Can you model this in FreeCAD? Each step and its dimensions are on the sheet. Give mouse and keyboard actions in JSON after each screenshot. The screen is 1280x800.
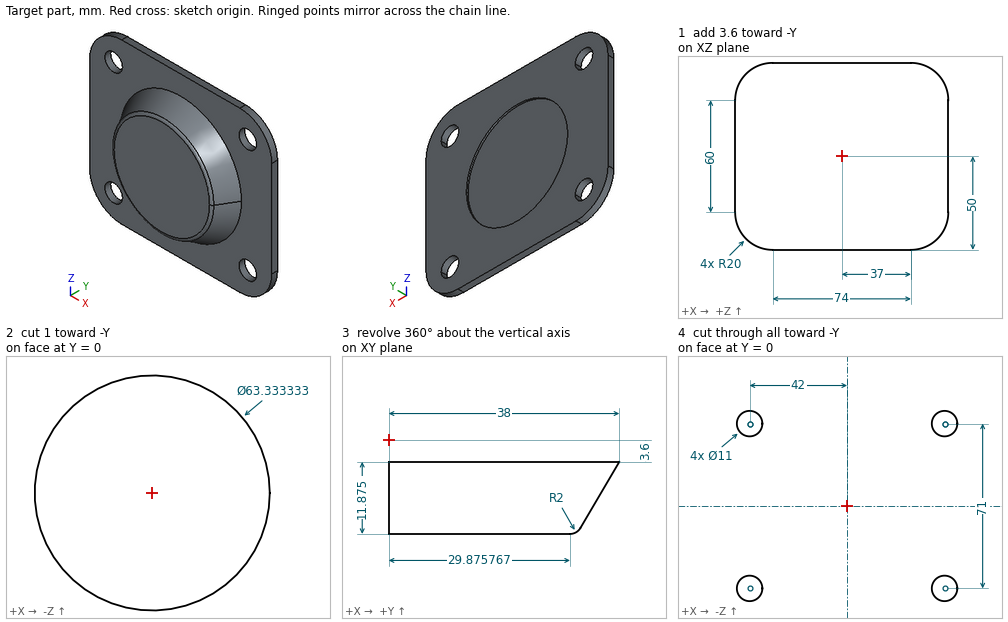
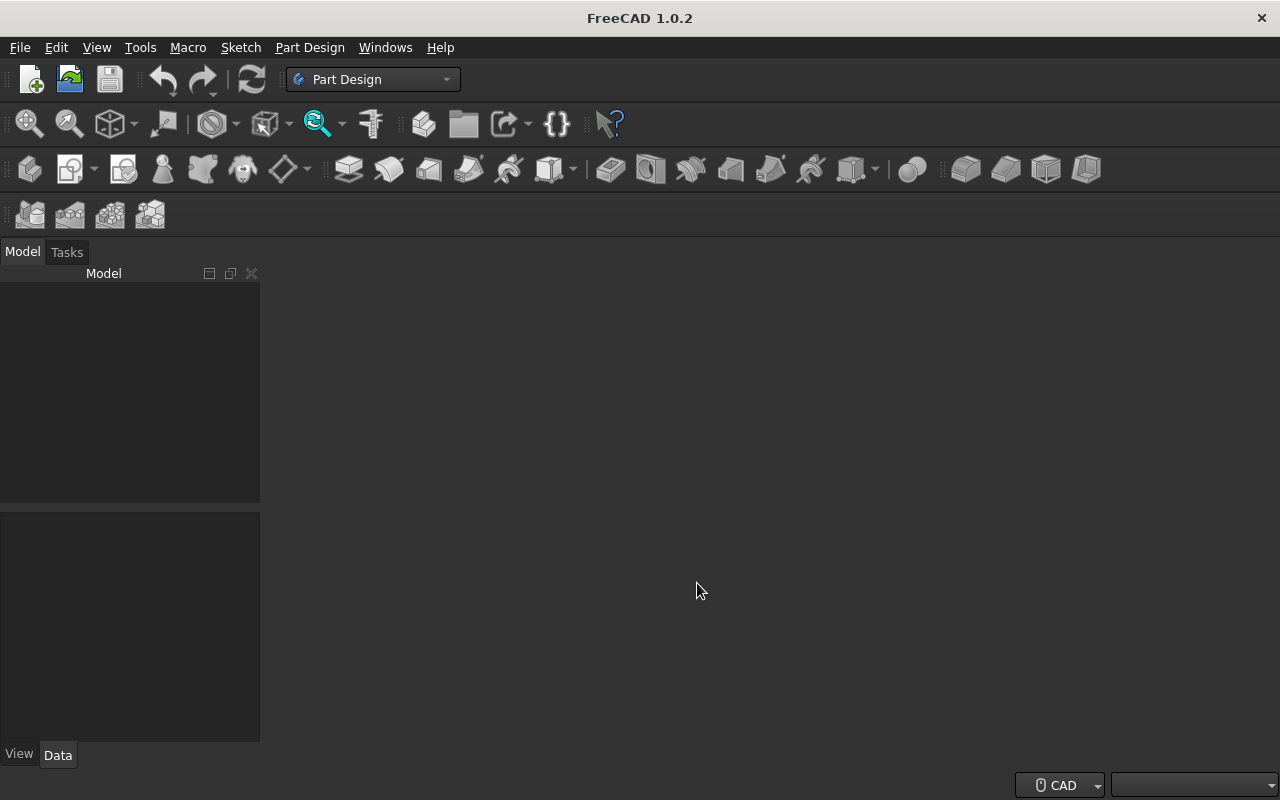
{"action": "left_click", "coordinate": [30, 80]}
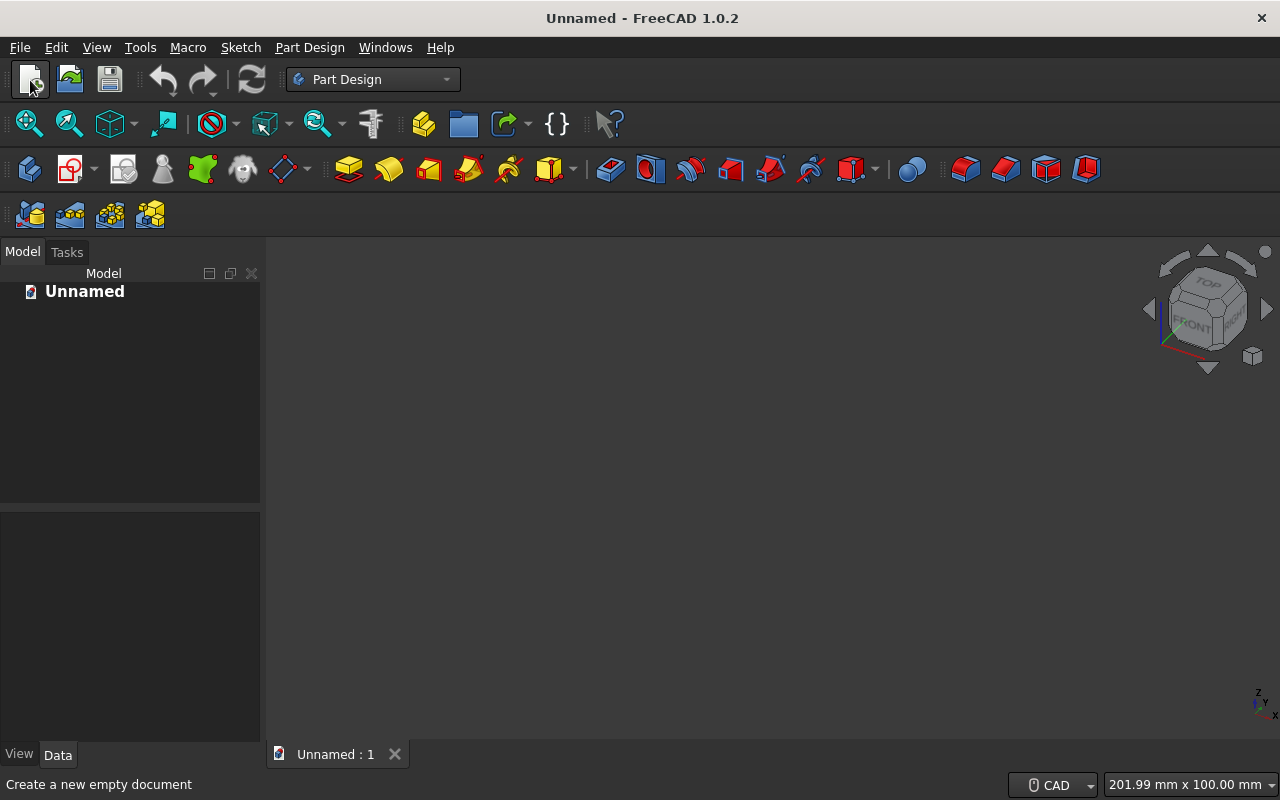
{"action": "left_click", "coordinate": [70, 170]}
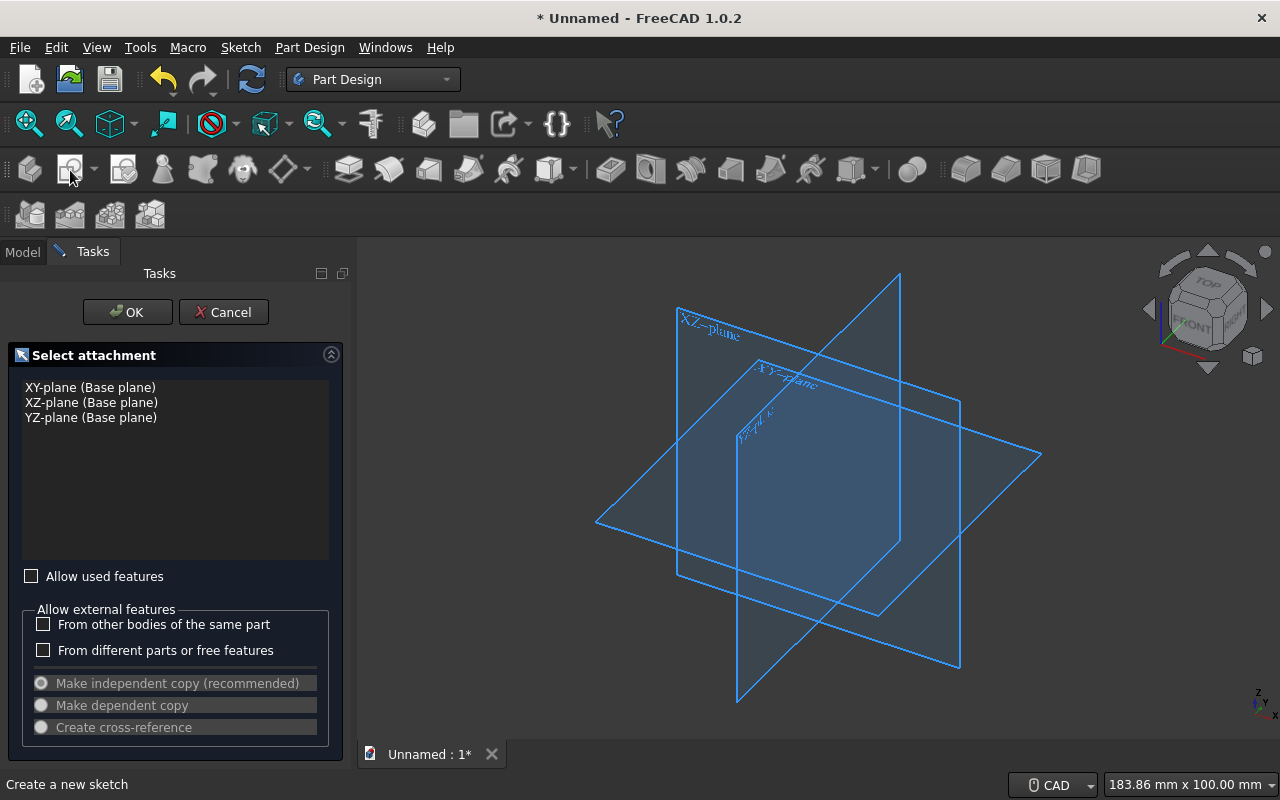
{"action": "left_click", "coordinate": [82, 402]}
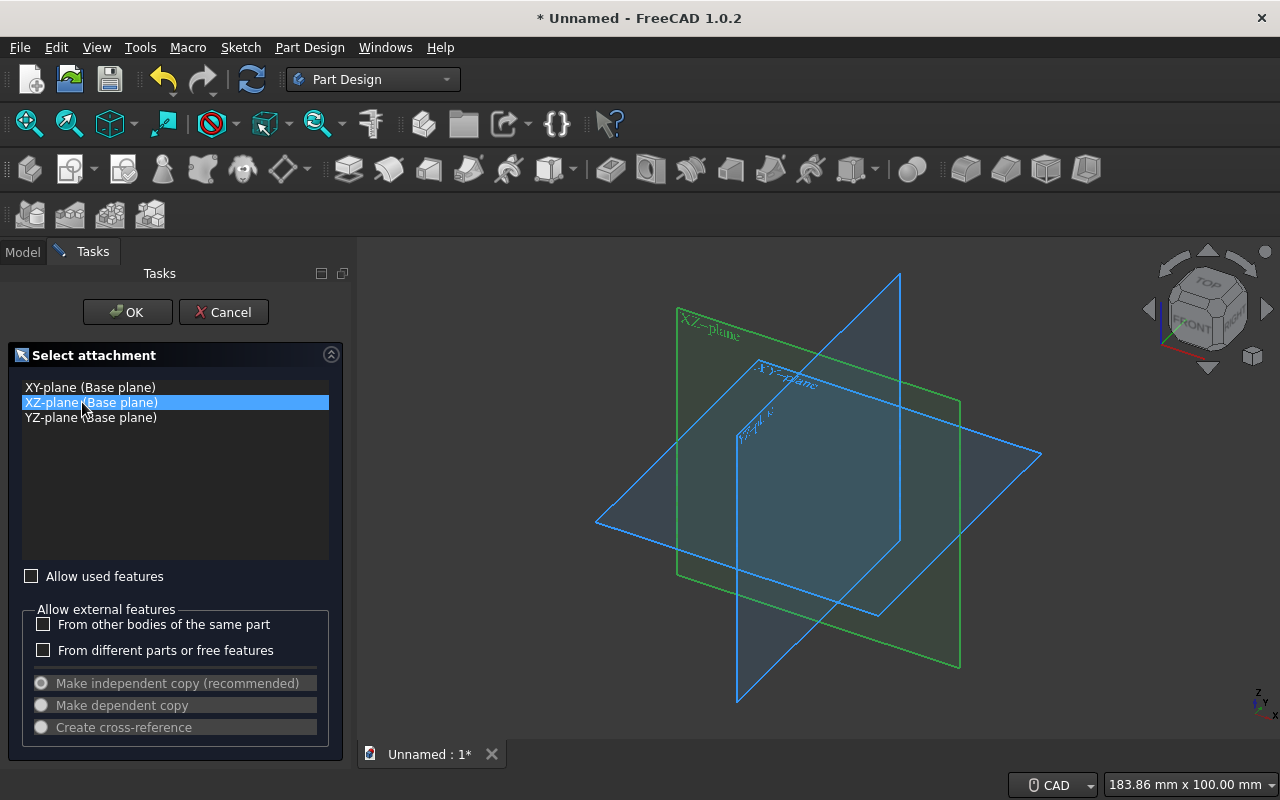
{"action": "left_click", "coordinate": [128, 312]}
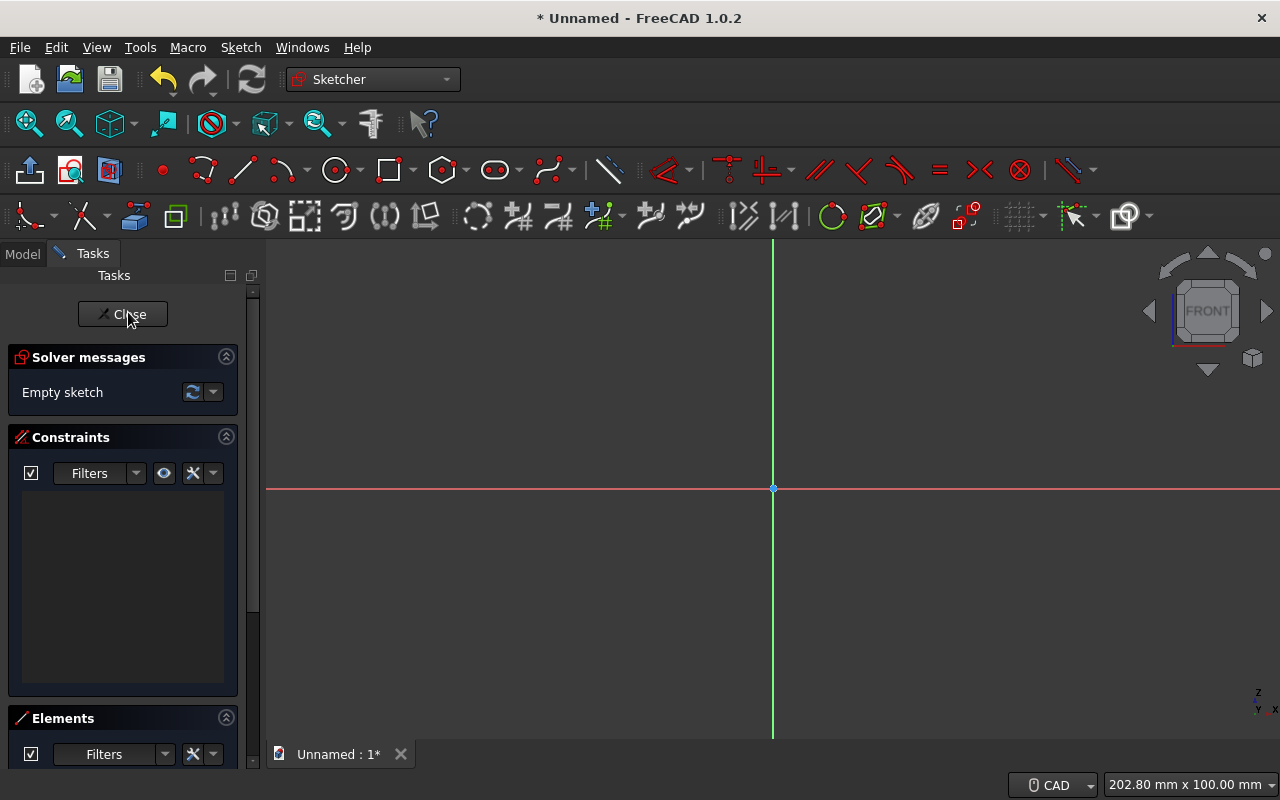
{"action": "scroll", "coordinate": [565, 489], "scroll_direction": "down", "scroll_amount": 2}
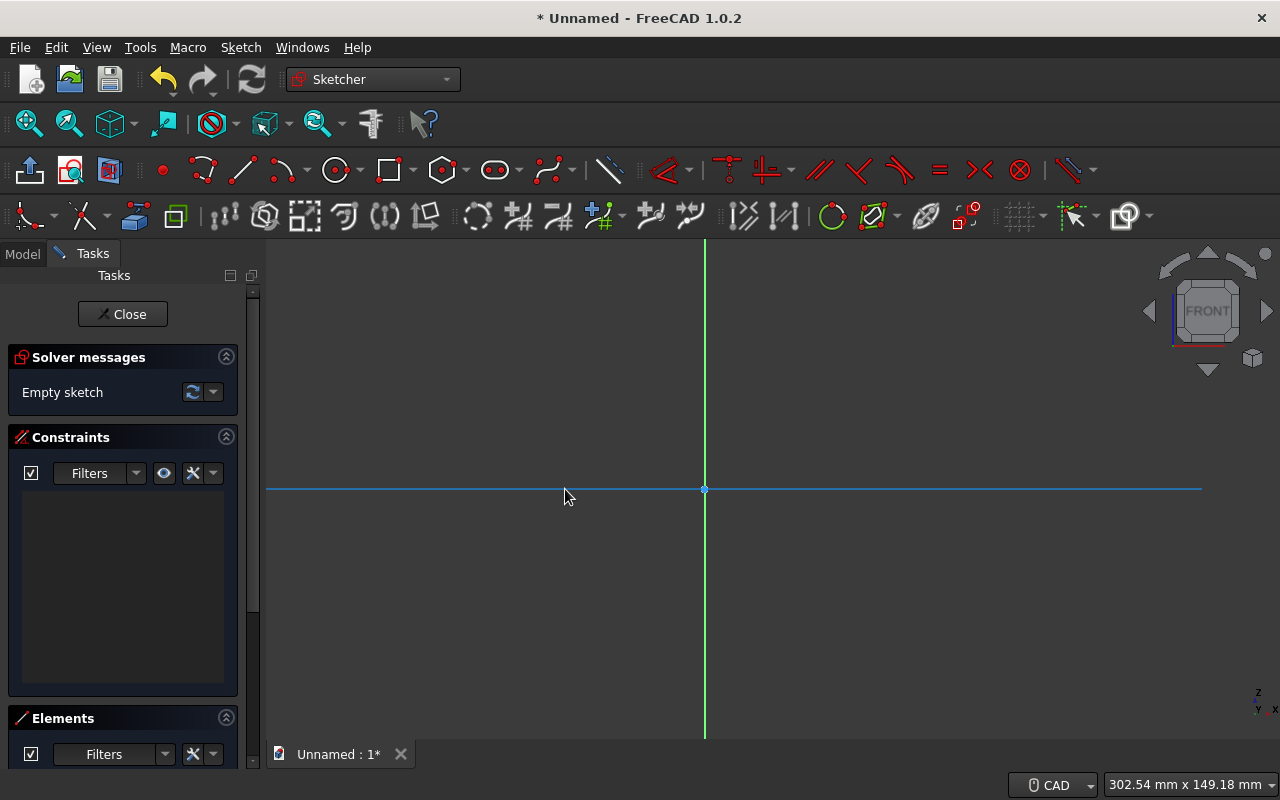
{"action": "left_click", "coordinate": [244, 170]}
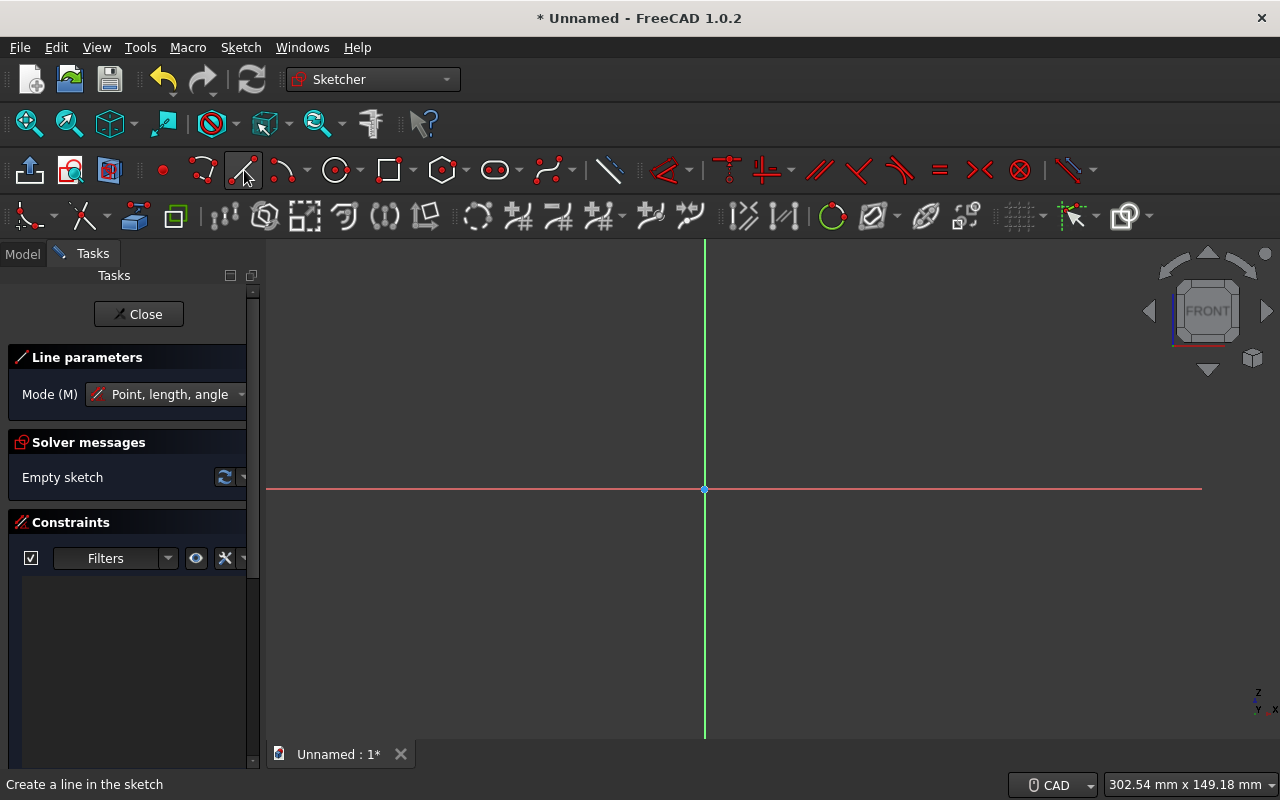
{"action": "left_click", "coordinate": [829, 657]}
{"action": "left_click", "coordinate": [581, 657]}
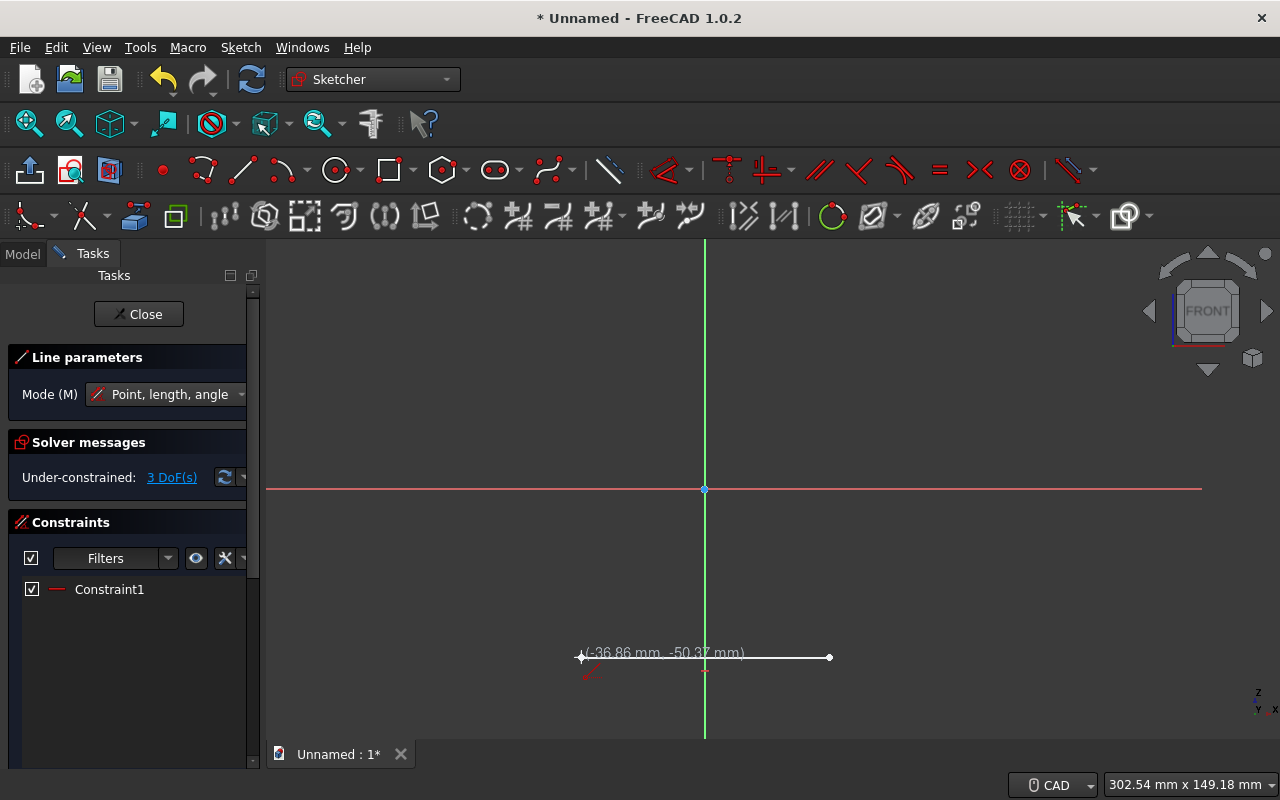
{"action": "left_click", "coordinate": [513, 590]}
{"action": "left_click", "coordinate": [513, 389]}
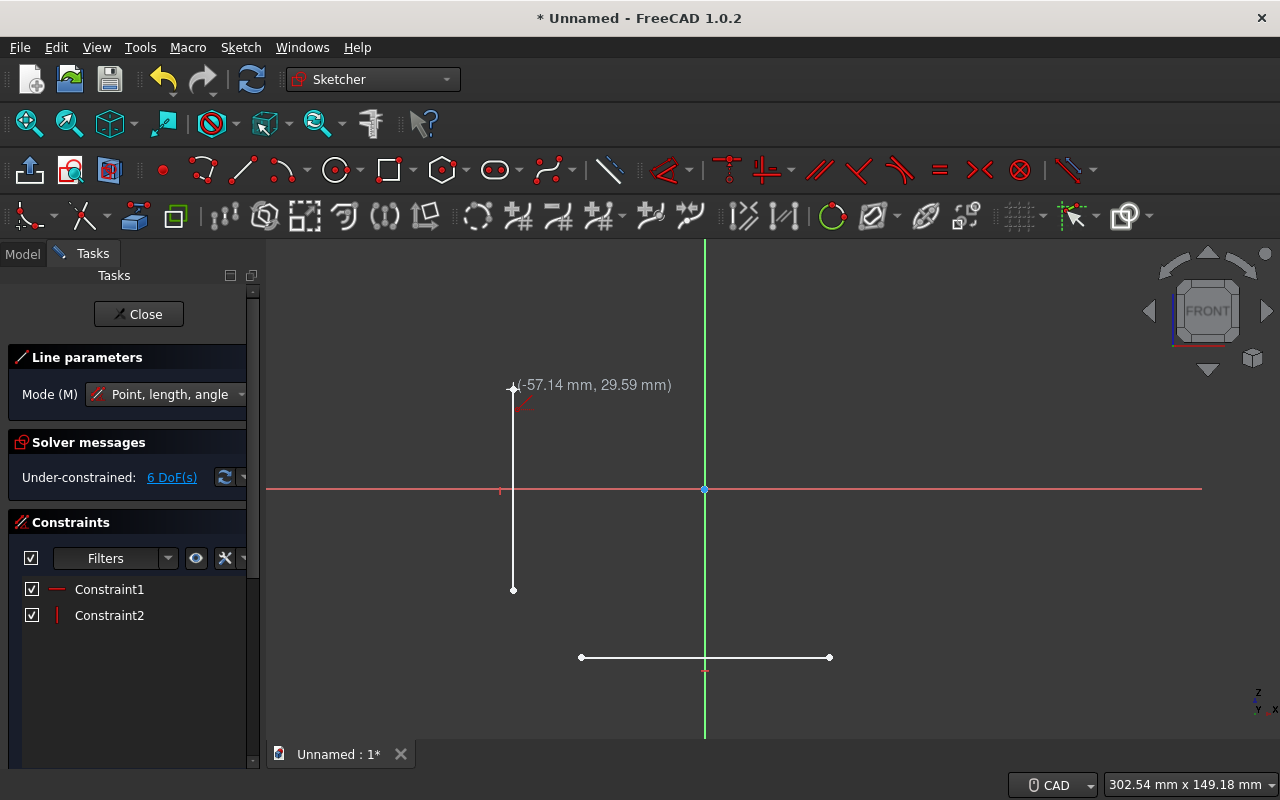
{"action": "left_click", "coordinate": [581, 322]}
{"action": "left_click", "coordinate": [829, 322]}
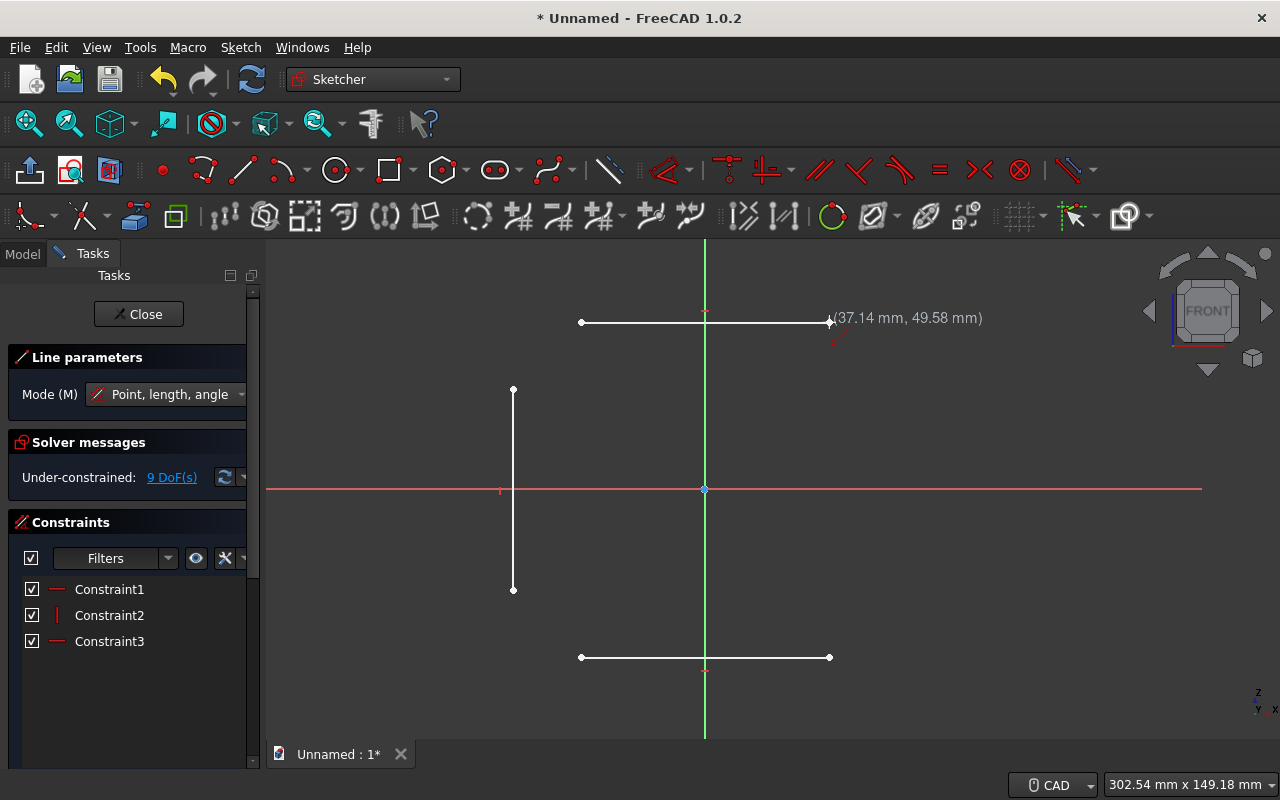
{"action": "left_click", "coordinate": [896, 389]}
{"action": "left_click", "coordinate": [896, 590]}